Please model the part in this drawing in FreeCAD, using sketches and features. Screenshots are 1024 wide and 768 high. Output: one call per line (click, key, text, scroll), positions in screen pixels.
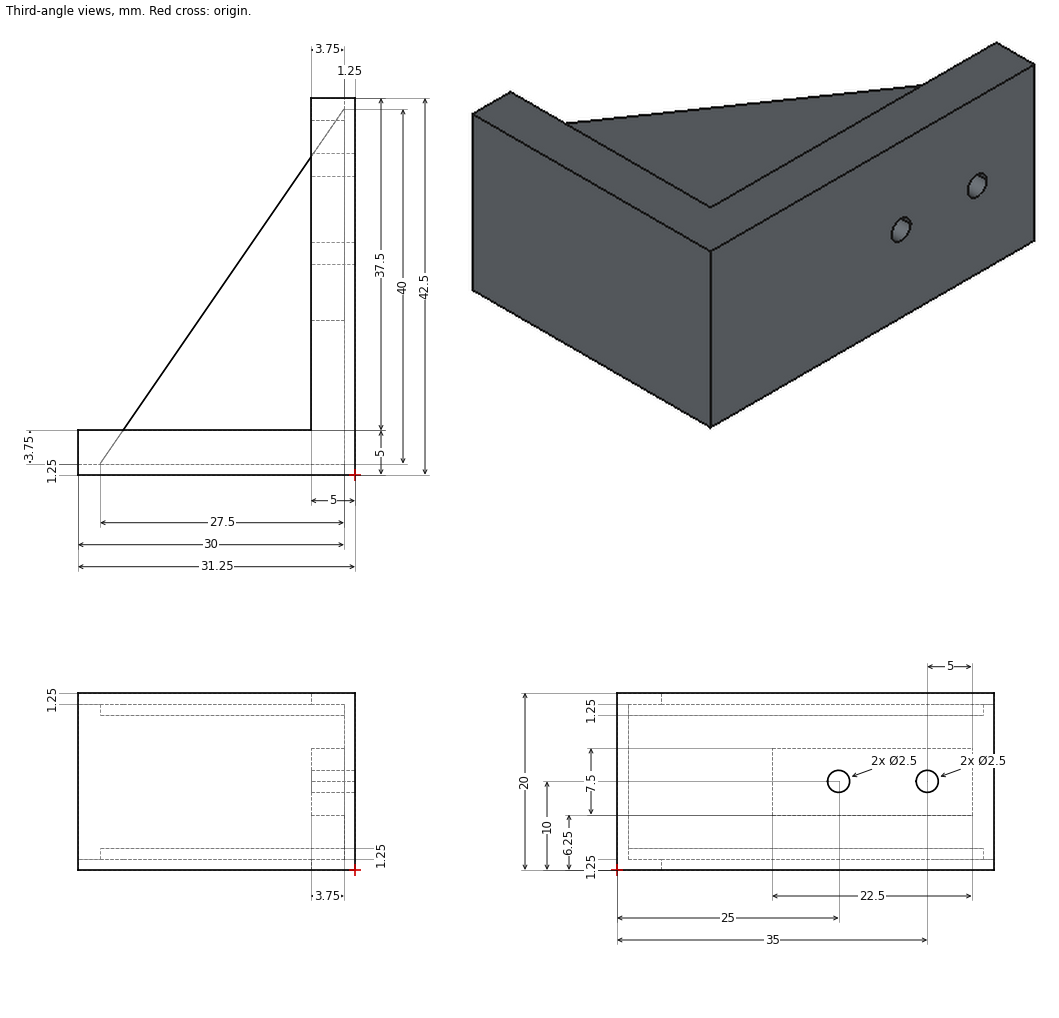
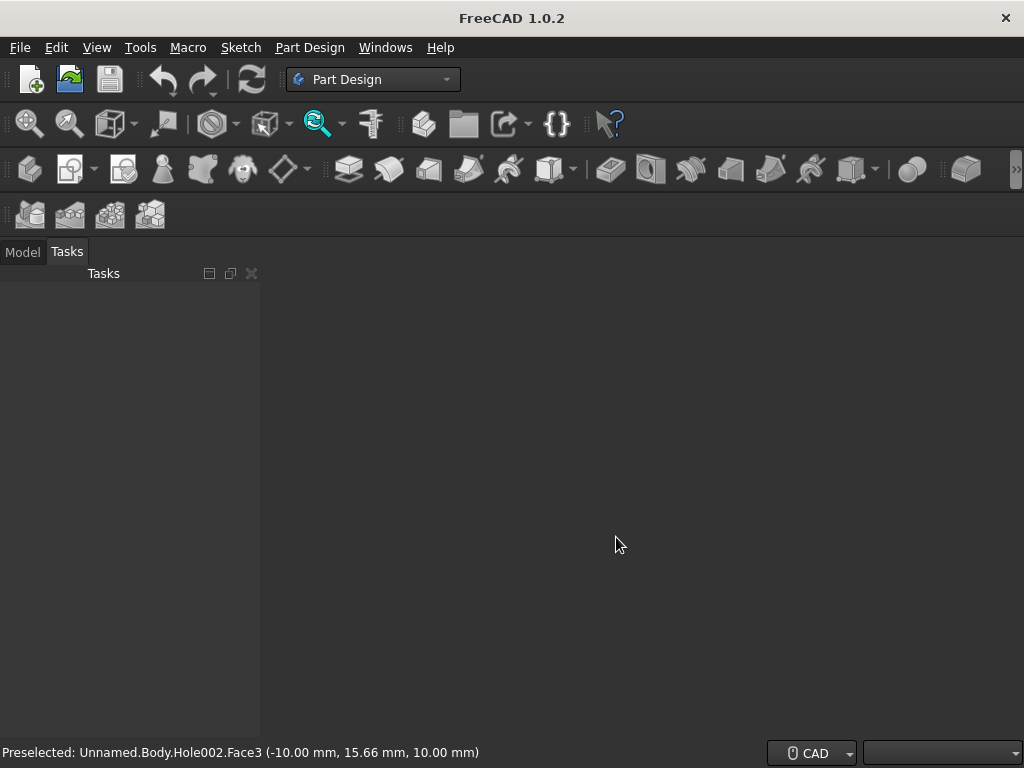
click(30, 80)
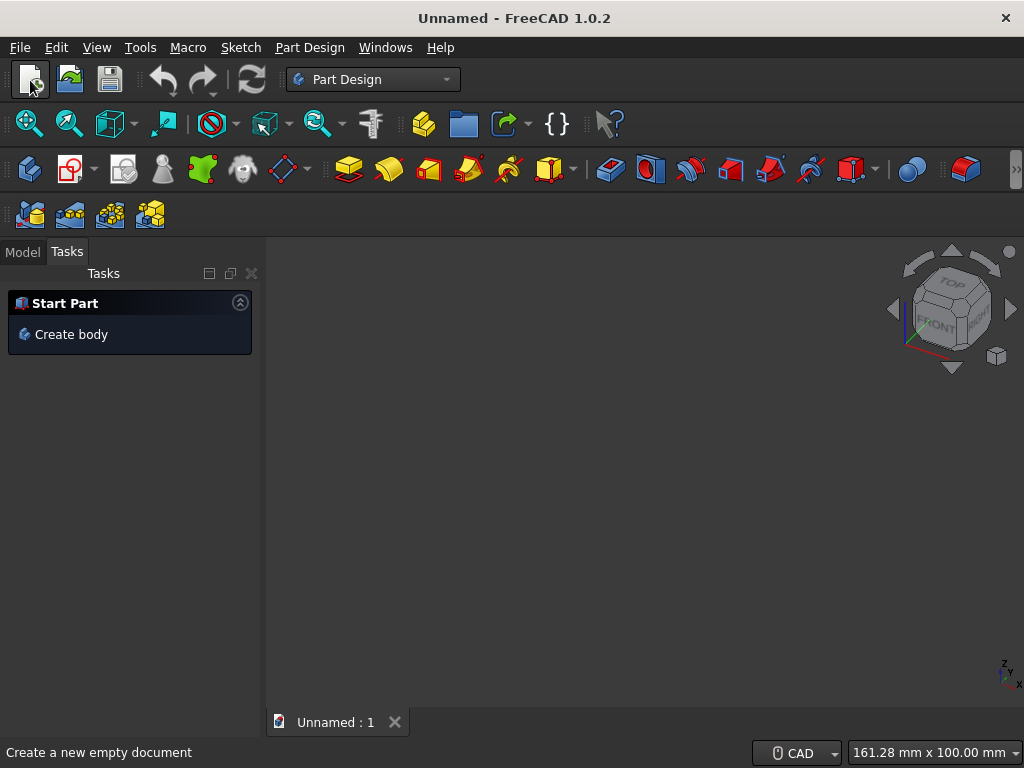
click(70, 170)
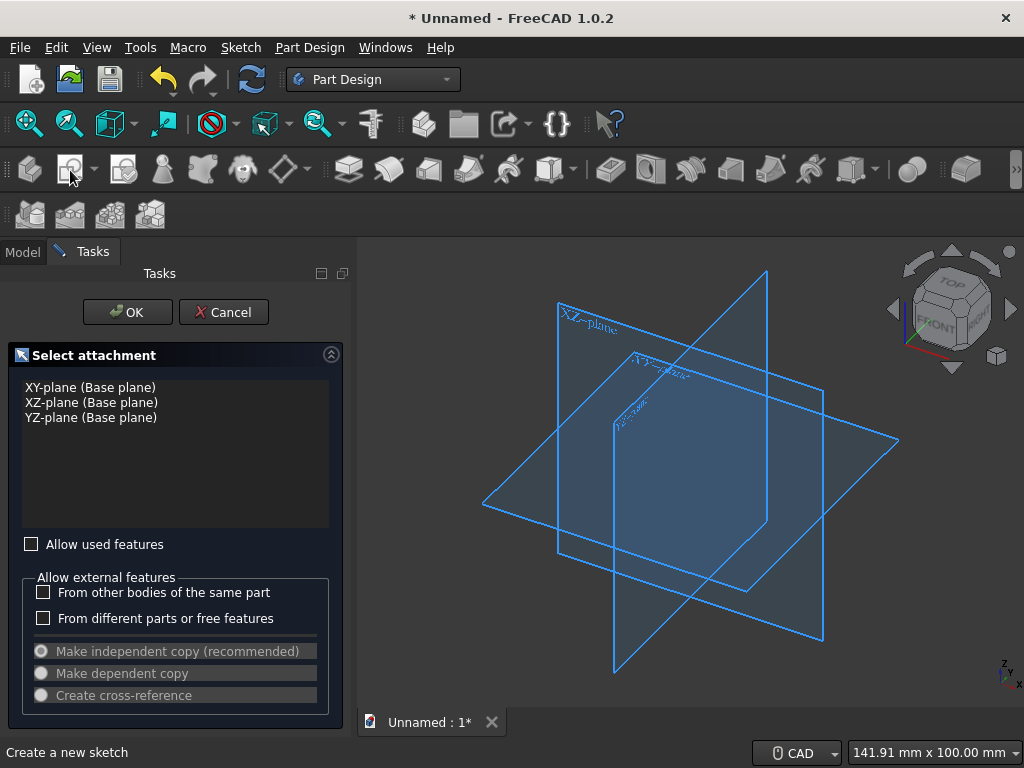
click(82, 388)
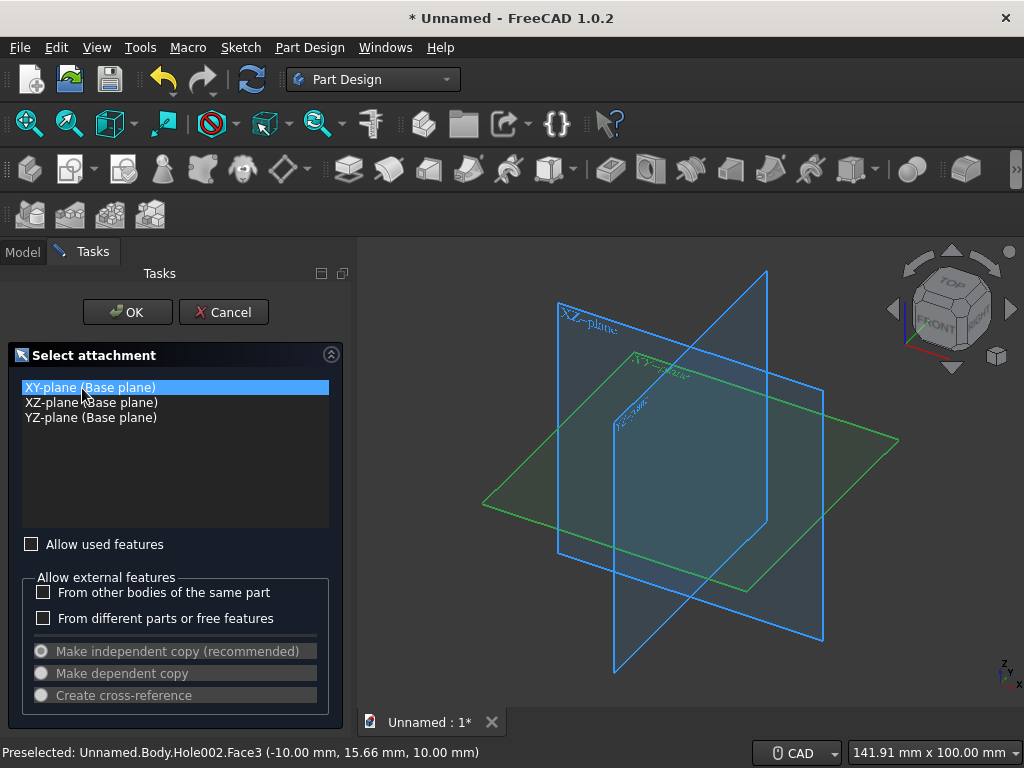
click(128, 312)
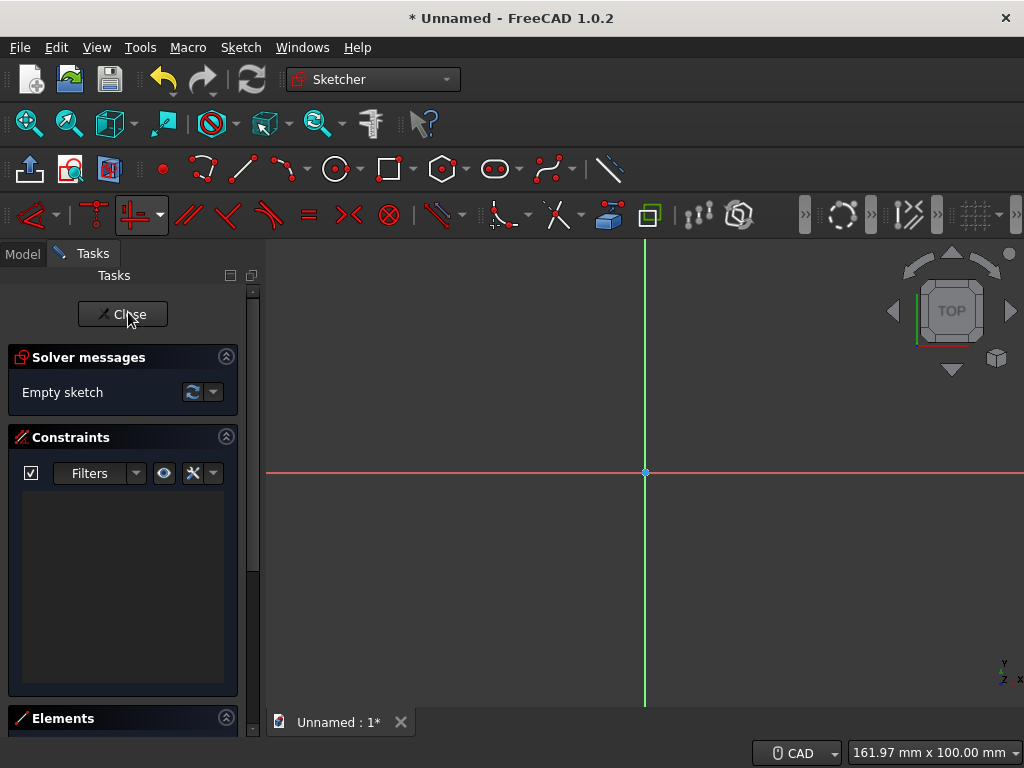
scroll(597, 679, down, 1)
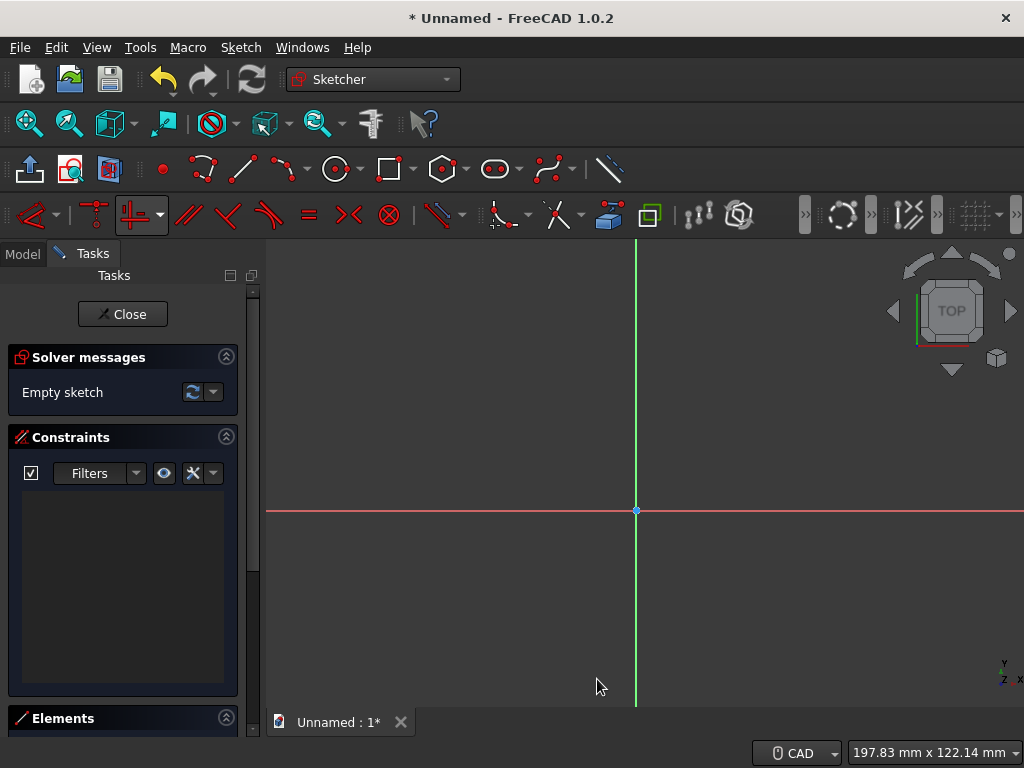
scroll(577, 376, up, 3)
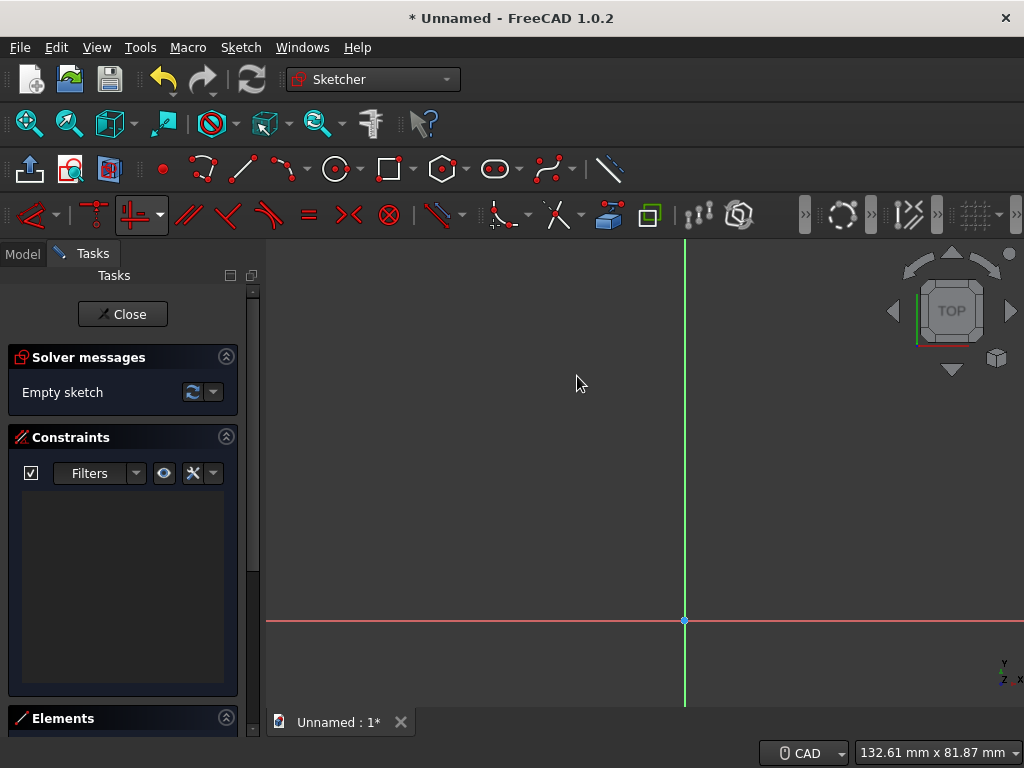
click(204, 170)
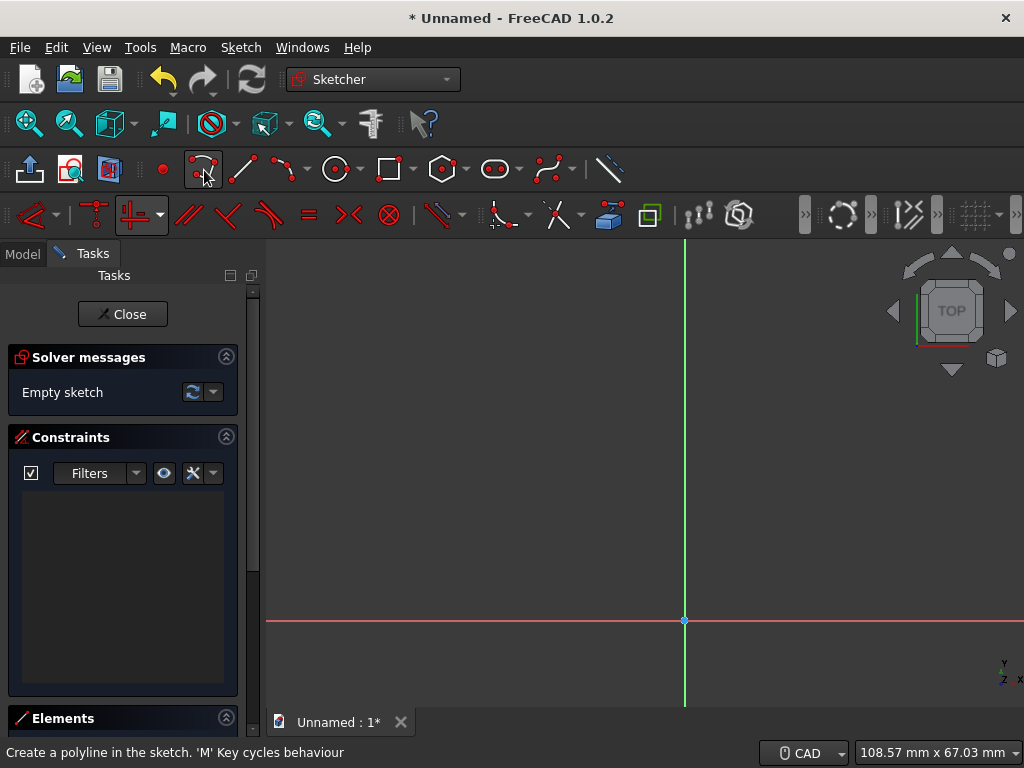
click(685, 621)
click(676, 324)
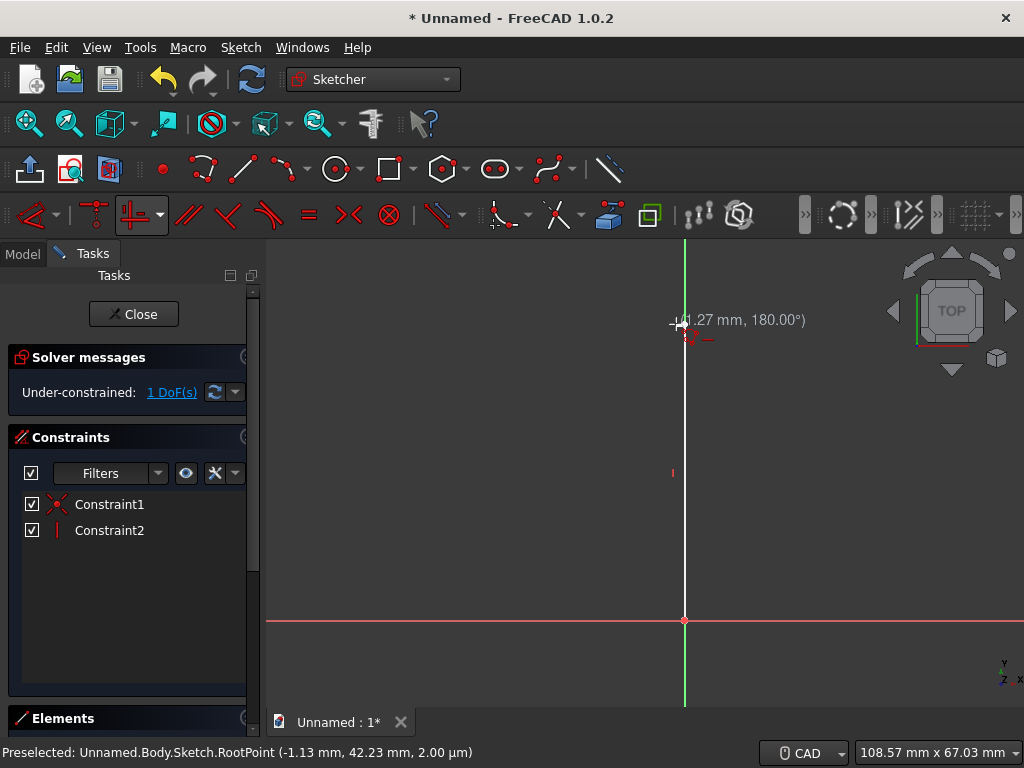
scroll(676, 324, up, 3)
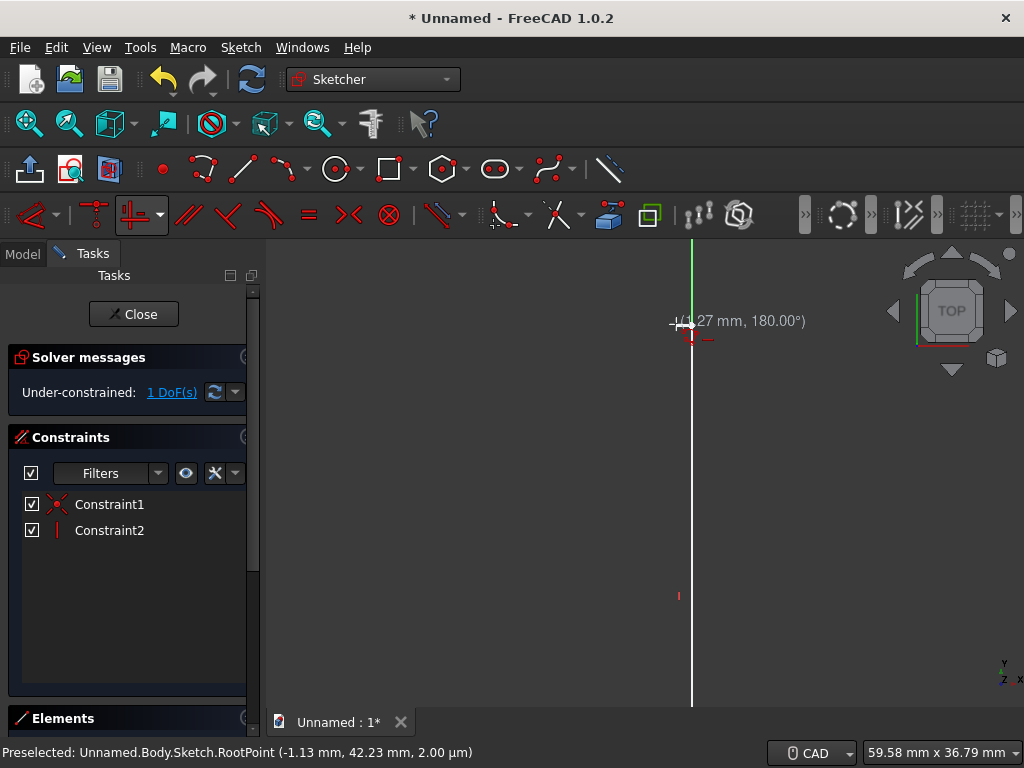
click(676, 324)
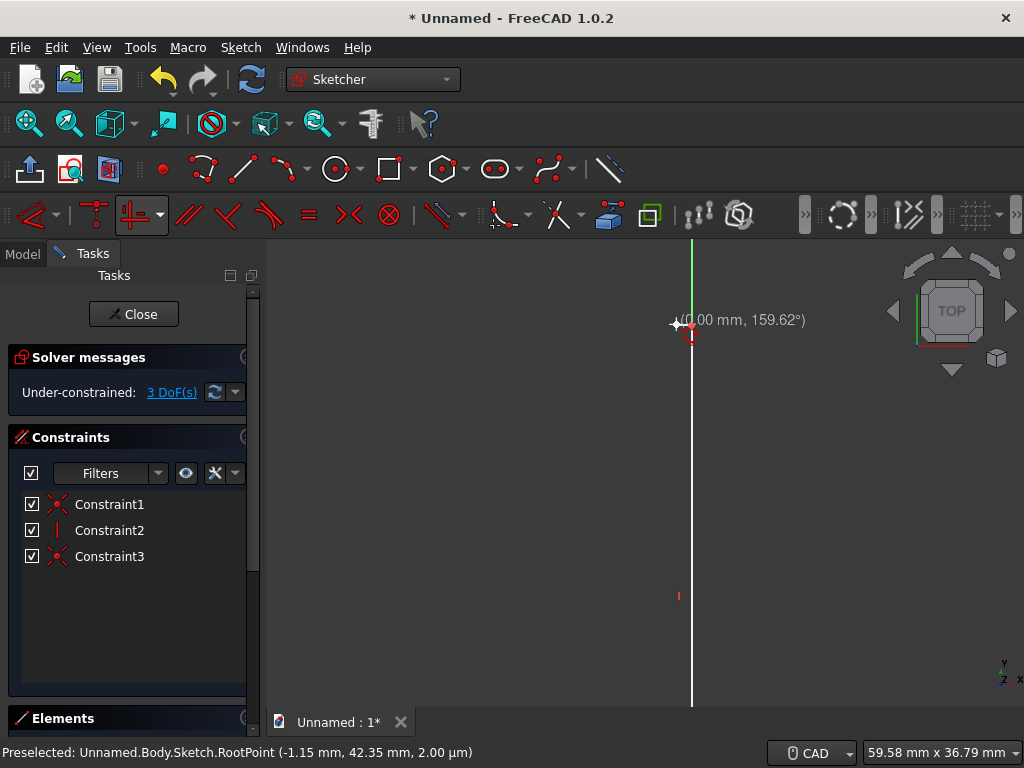
scroll(678, 325, down, 3)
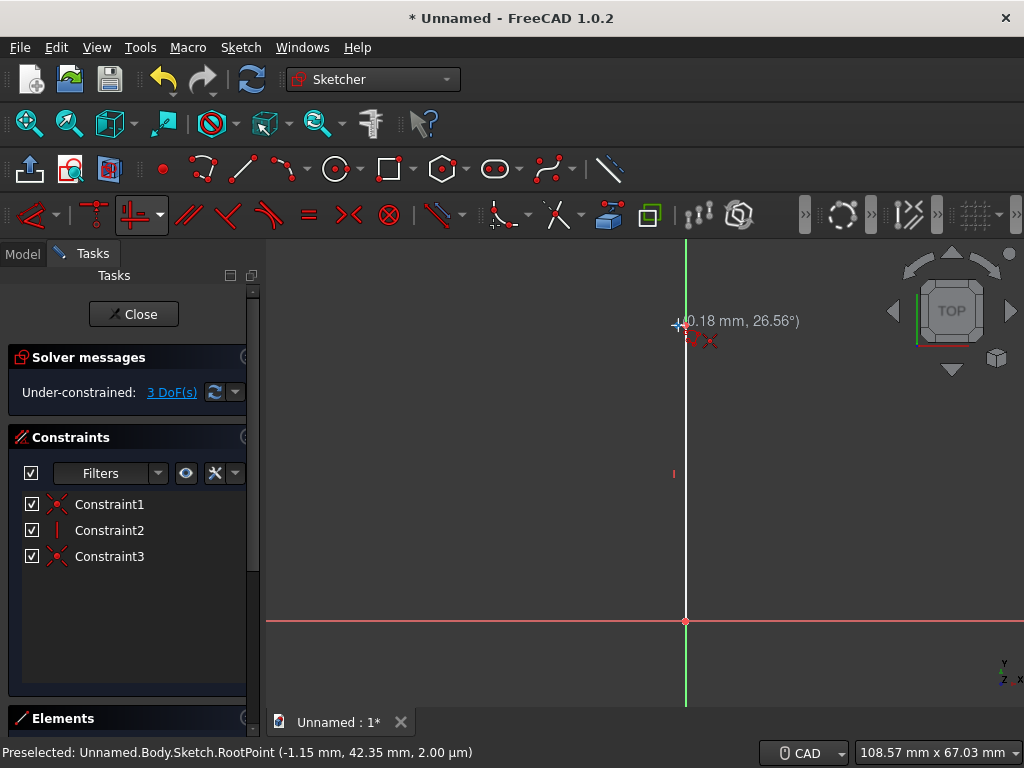
scroll(677, 613, up, 3)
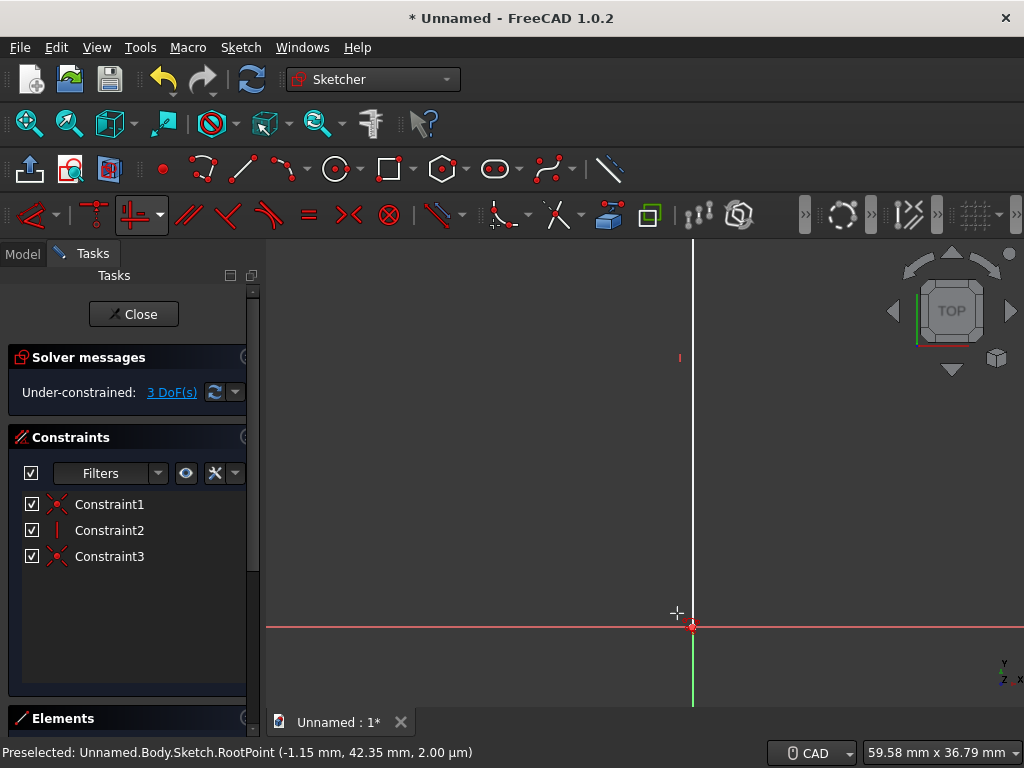
click(677, 612)
click(295, 612)
click(295, 618)
click(693, 627)
key(Escape)
key(Escape)